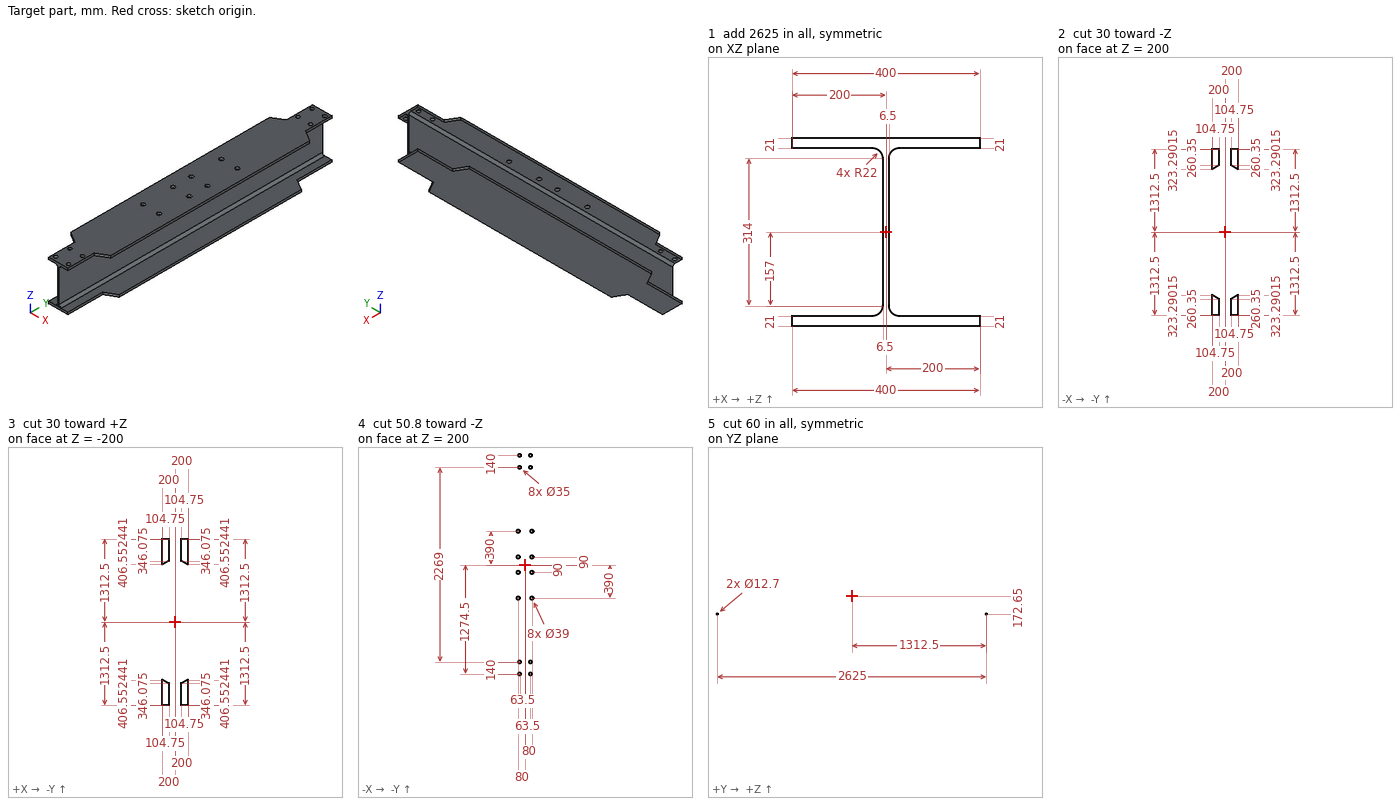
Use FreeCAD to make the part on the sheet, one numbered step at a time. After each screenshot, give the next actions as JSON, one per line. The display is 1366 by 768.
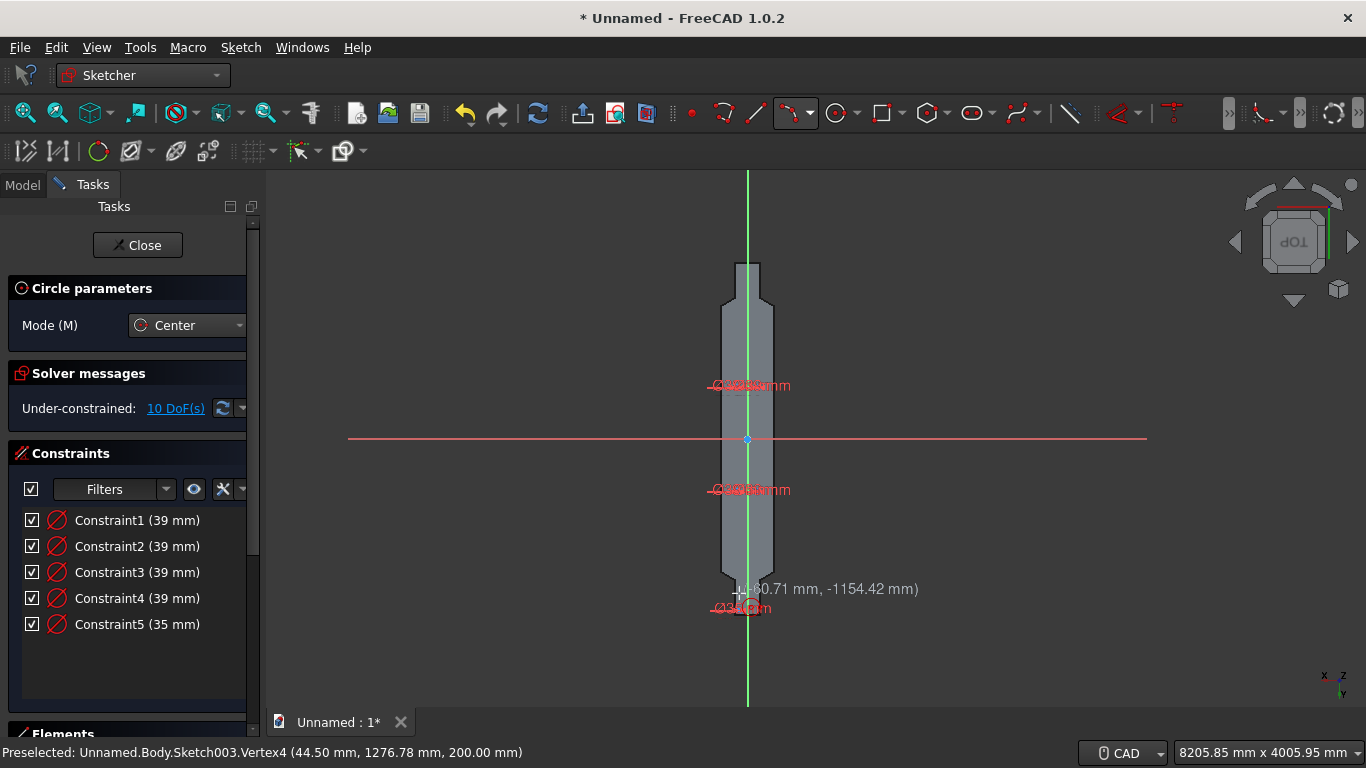
{"action": "scroll", "coordinate": [739, 591], "scroll_direction": "up", "scroll_amount": 4}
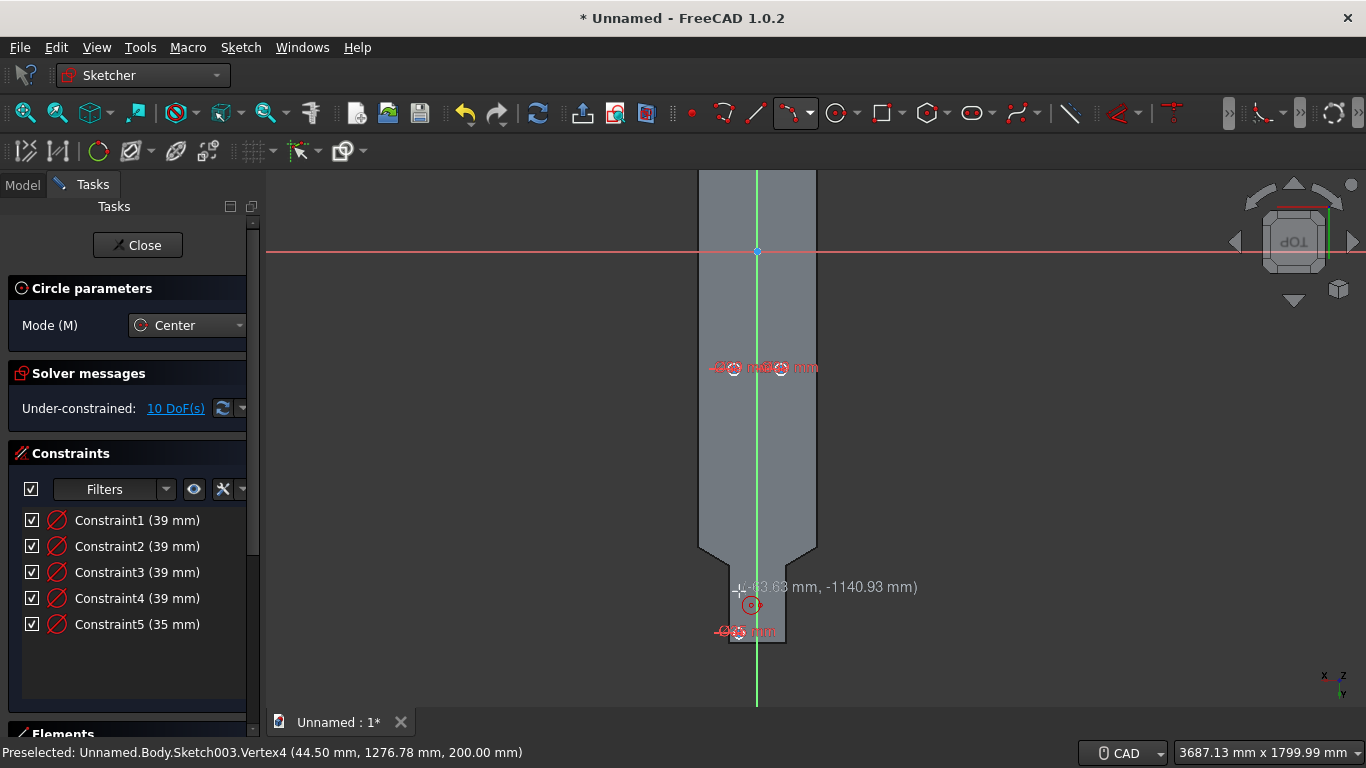
{"action": "left_click", "coordinate": [739, 590]}
{"action": "mouse_move", "coordinate": [742, 587]}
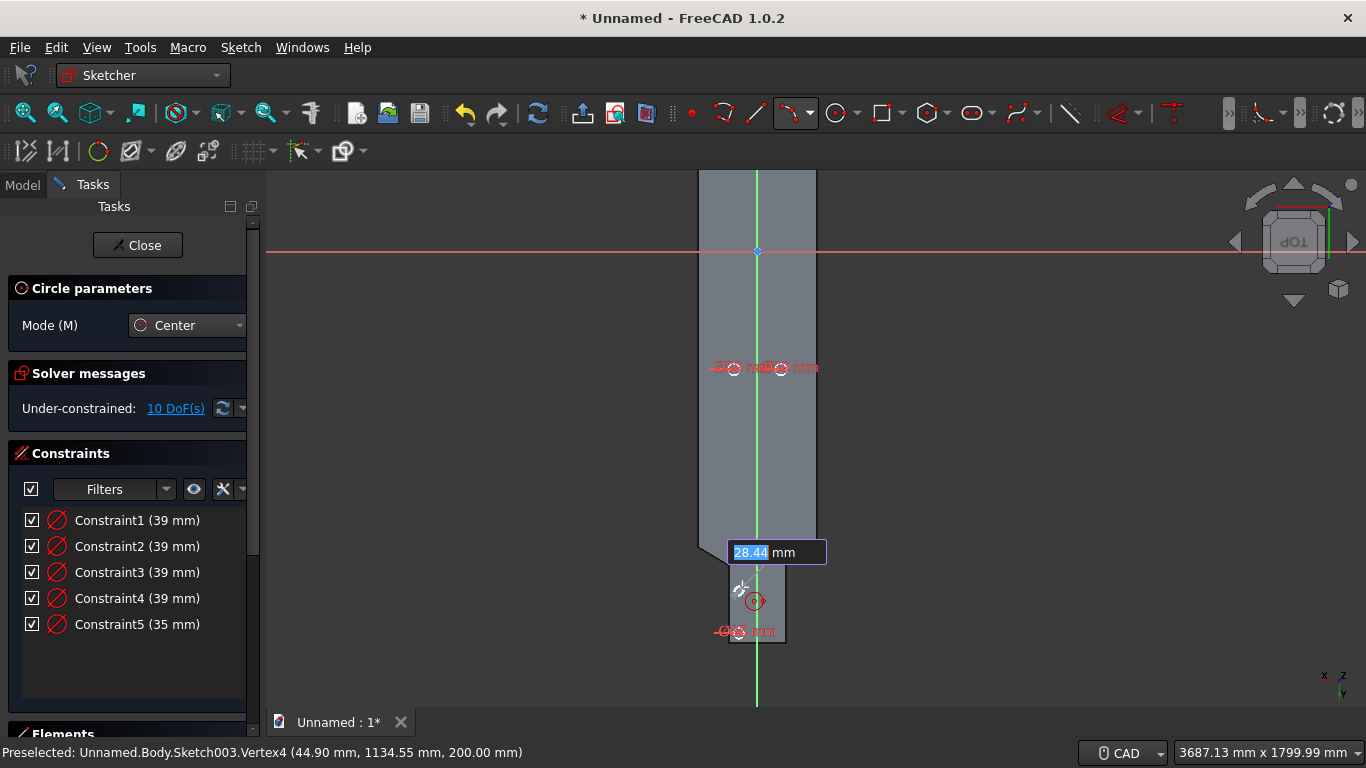
{"action": "type", "text": "35"}
{"action": "key", "text": "Return"}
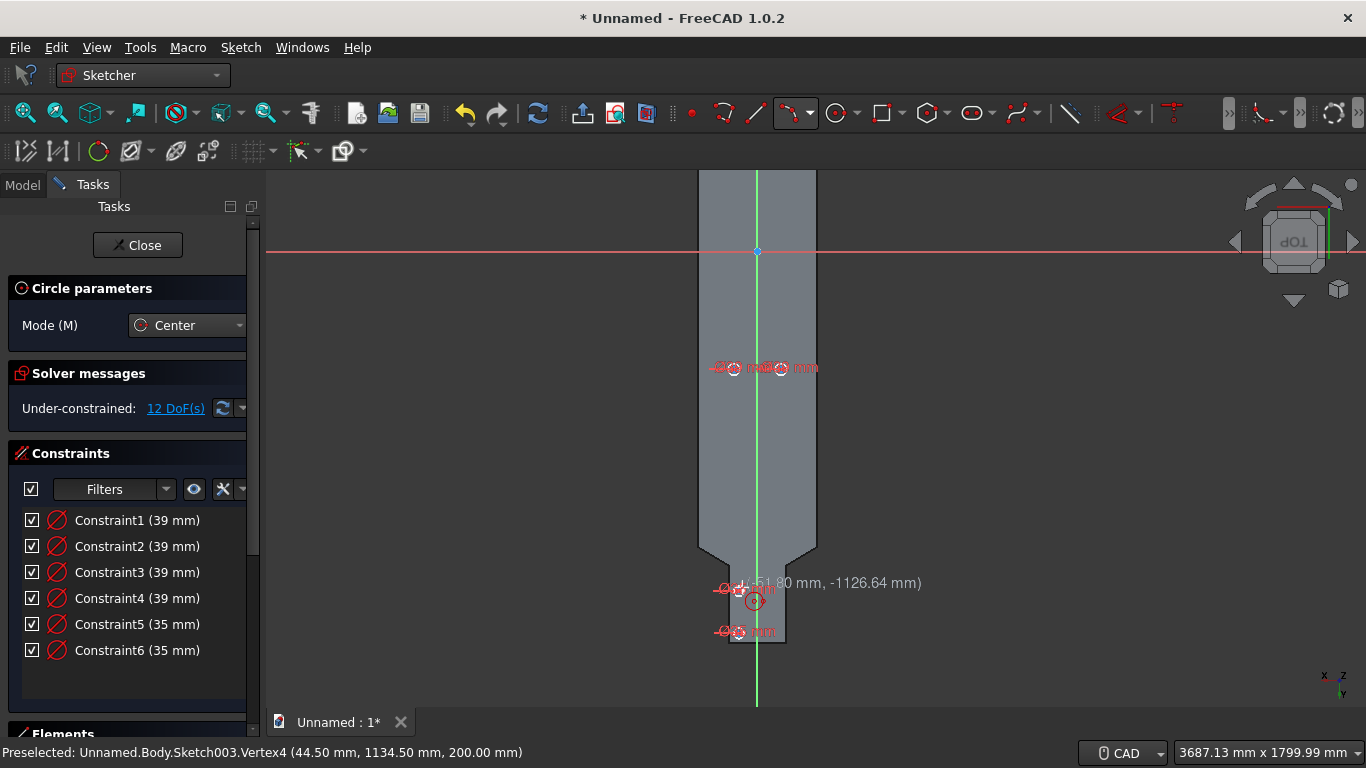
{"action": "scroll", "coordinate": [776, 632], "scroll_direction": "up", "scroll_amount": 8}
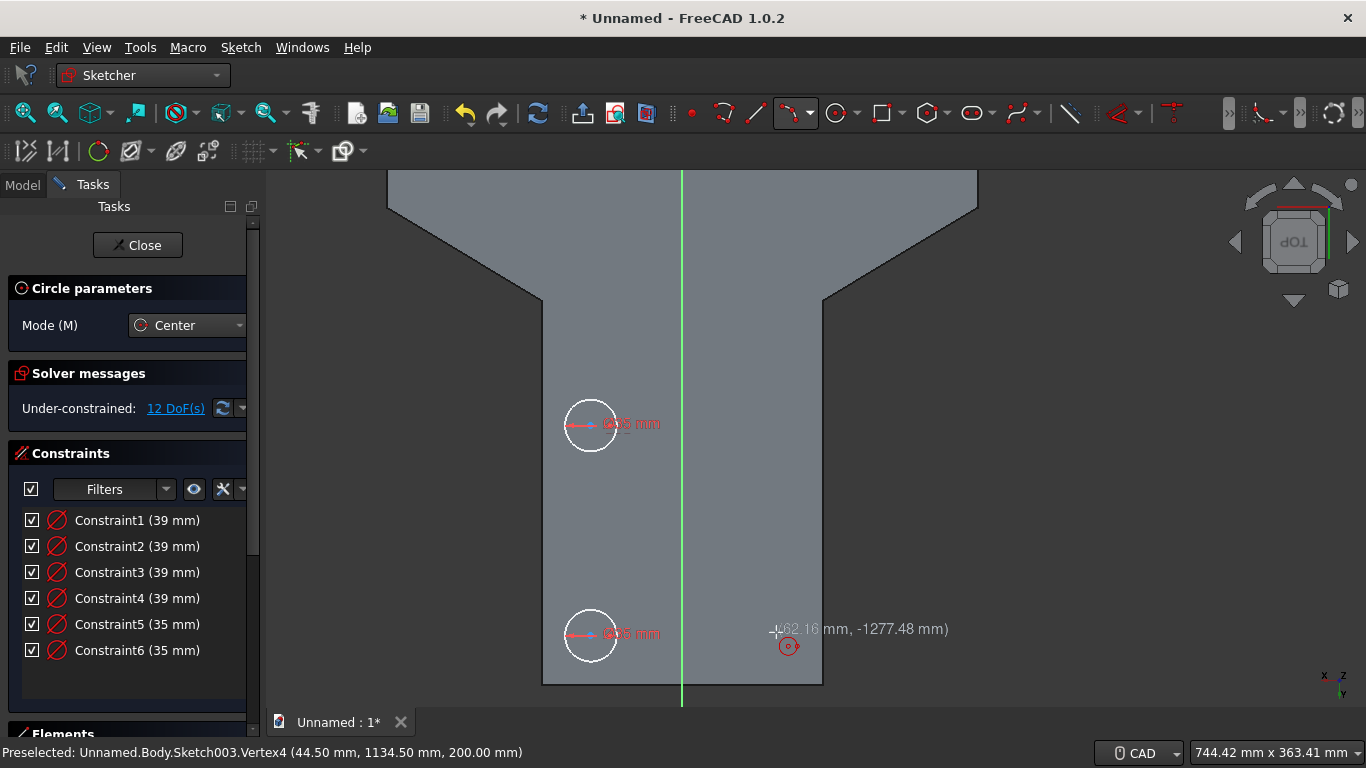
{"action": "scroll", "coordinate": [754, 607], "scroll_direction": "down", "scroll_amount": 12}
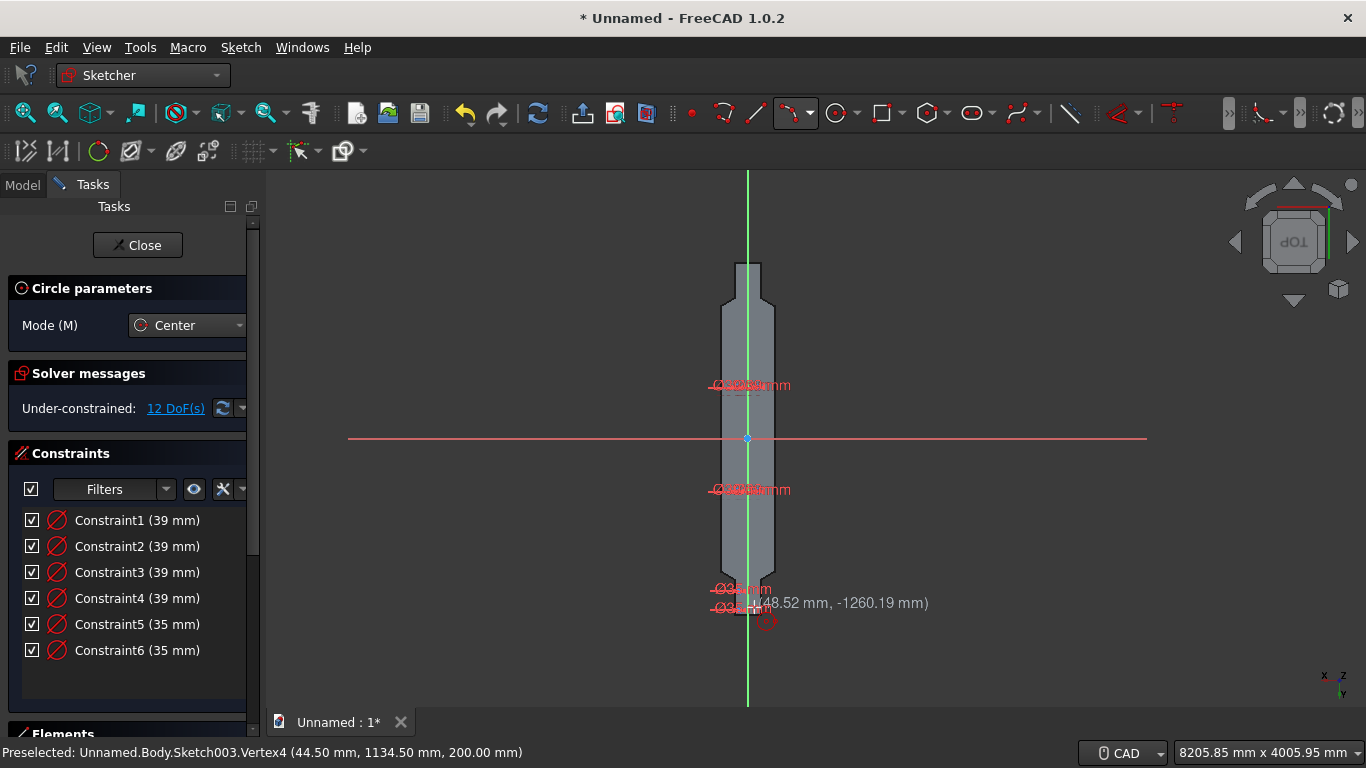
{"action": "scroll", "coordinate": [756, 610], "scroll_direction": "up", "scroll_amount": 4}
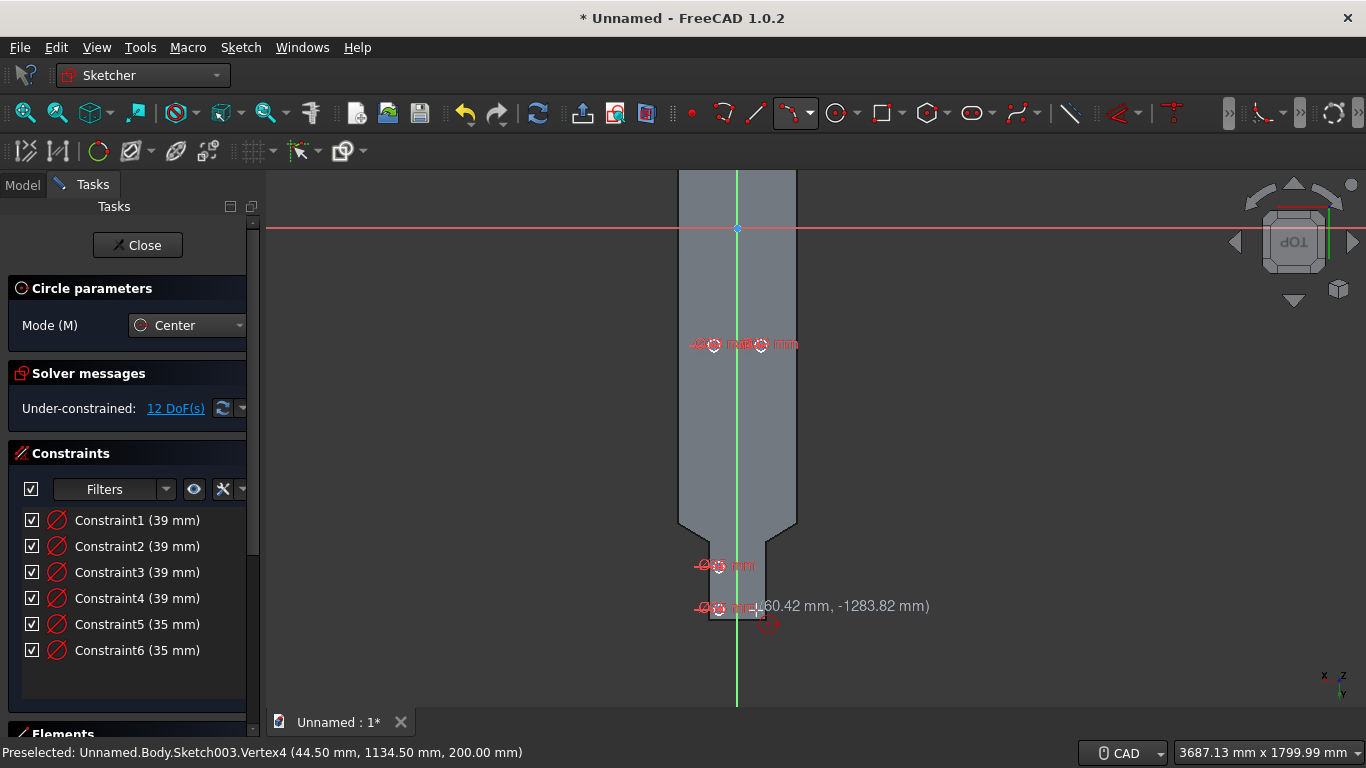
{"action": "left_click", "coordinate": [756, 608]}
{"action": "mouse_move", "coordinate": [760, 605]}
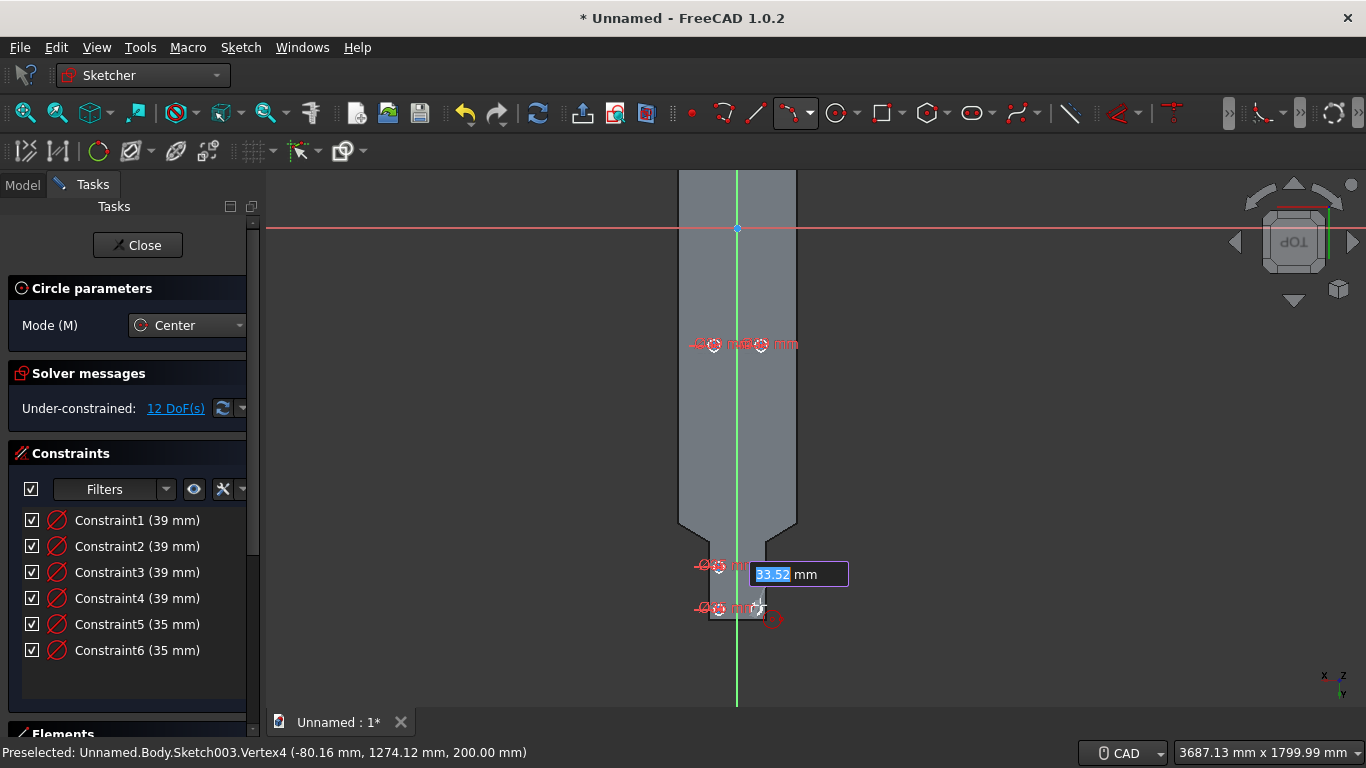
{"action": "type", "text": "35"}
{"action": "key", "text": "Return"}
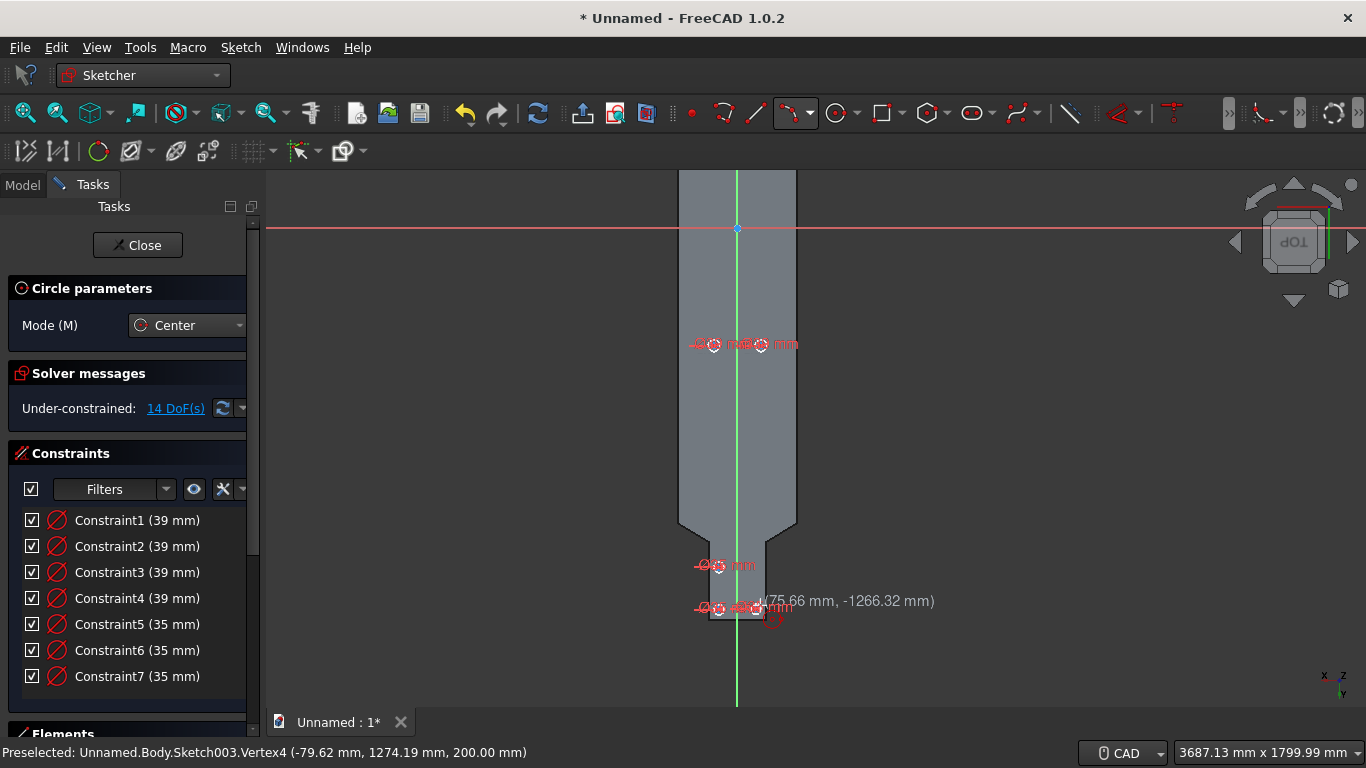
{"action": "scroll", "coordinate": [756, 567], "scroll_direction": "up", "scroll_amount": 8}